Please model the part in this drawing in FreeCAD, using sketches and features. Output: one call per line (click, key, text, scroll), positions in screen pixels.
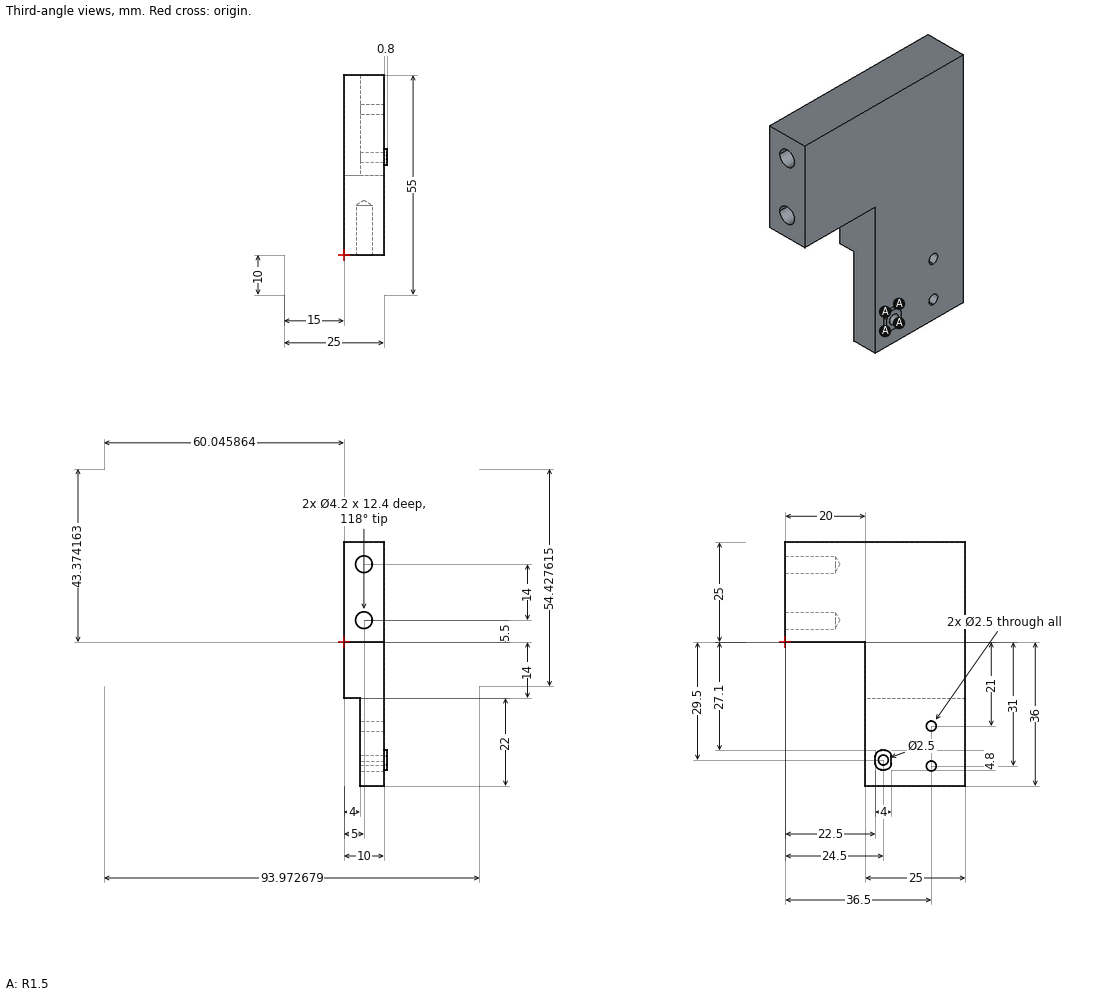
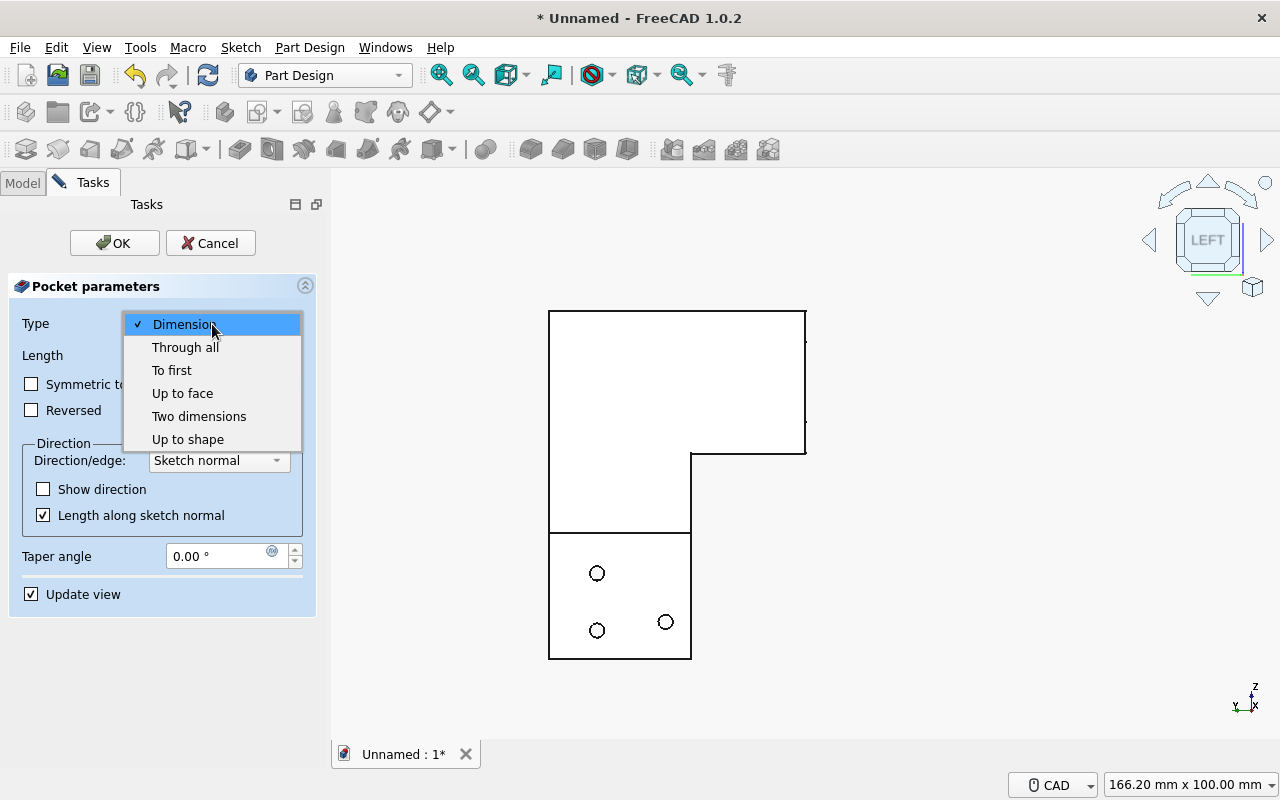
click(212, 348)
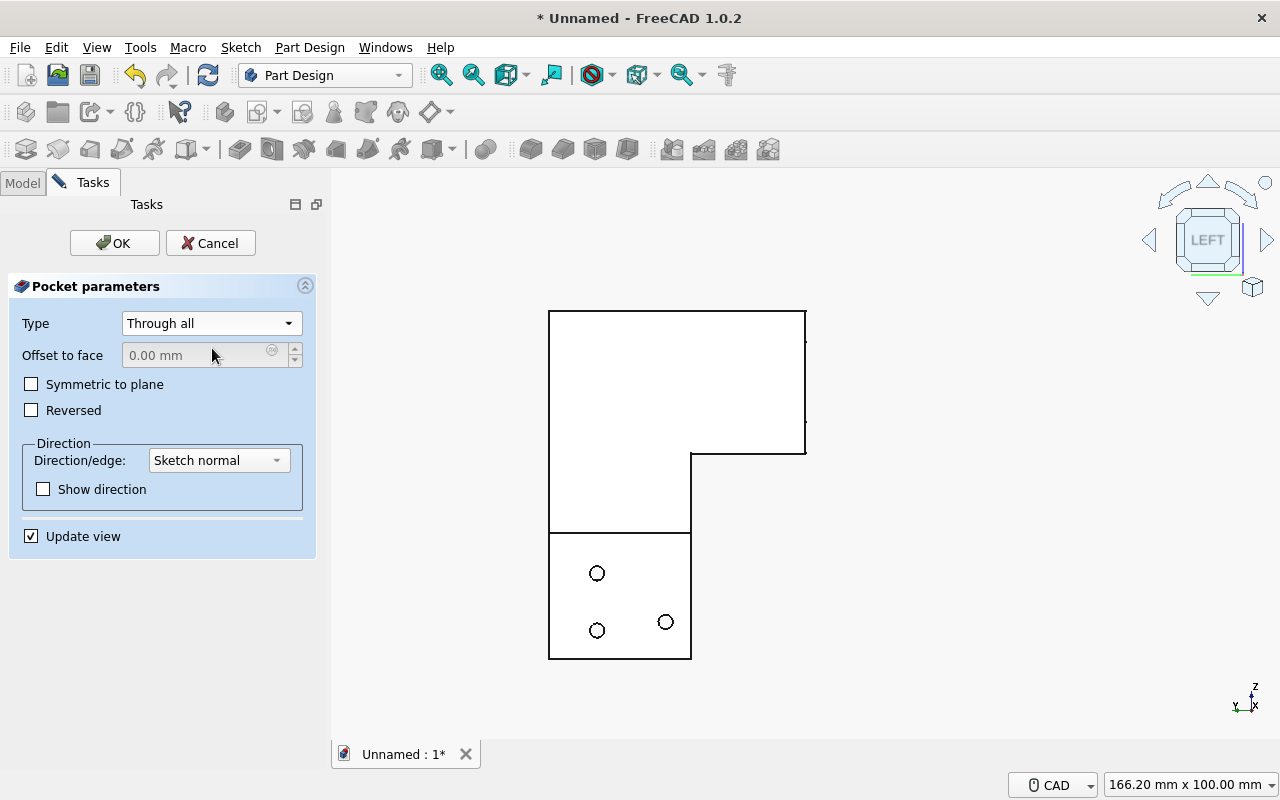
click(115, 243)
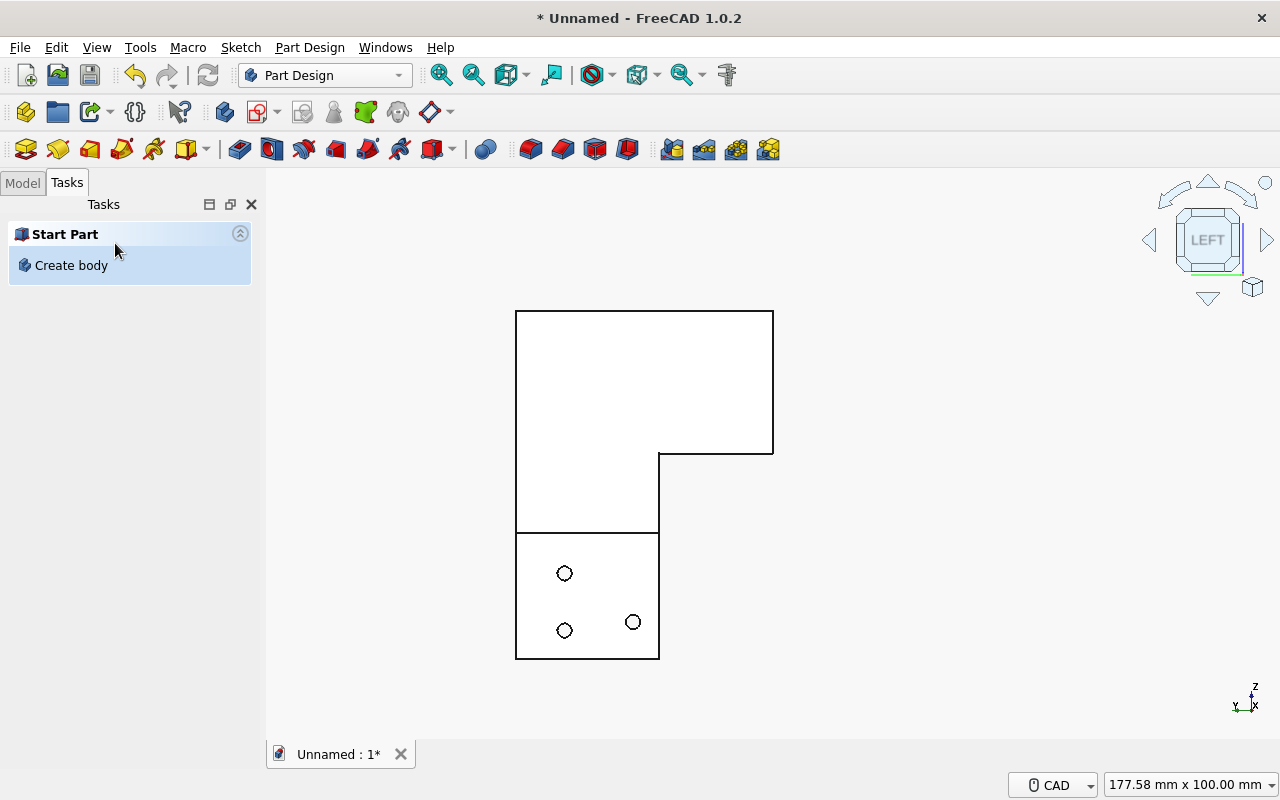
scroll(645, 635, up, 11)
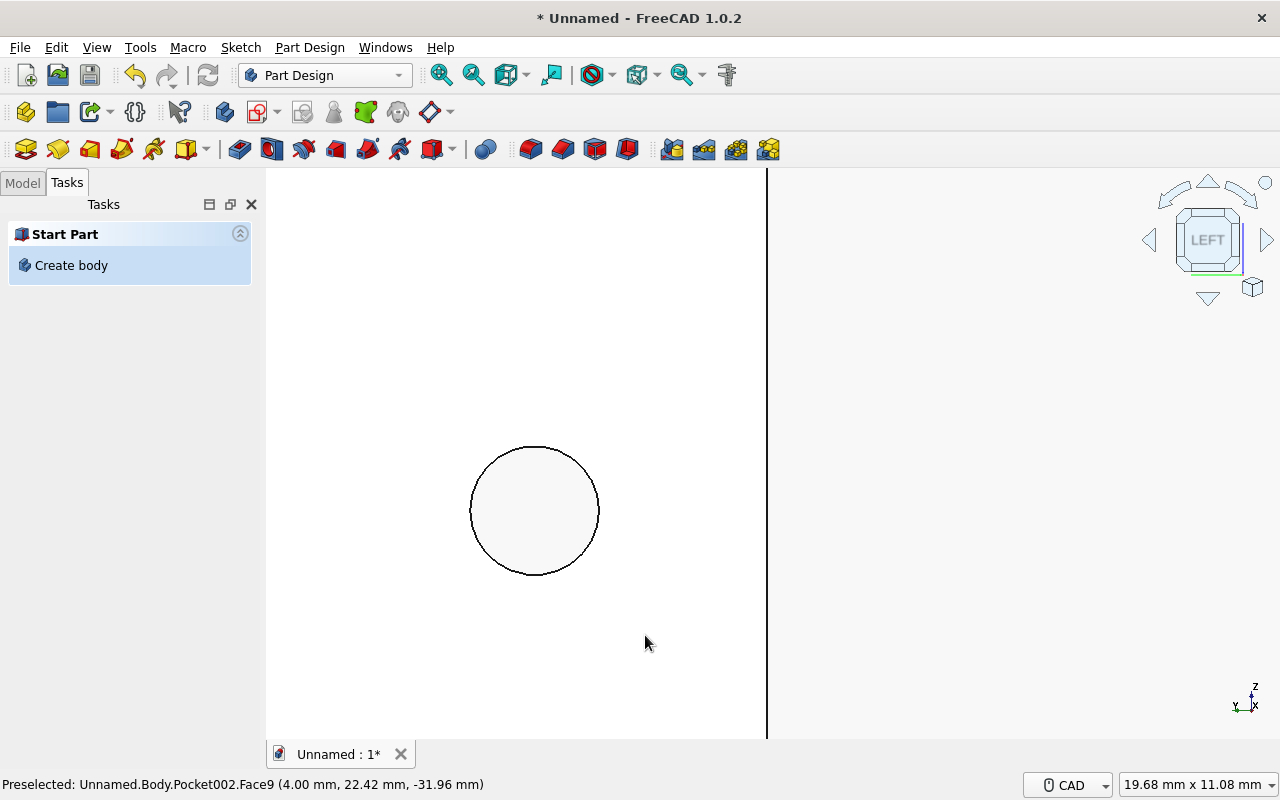
click(442, 76)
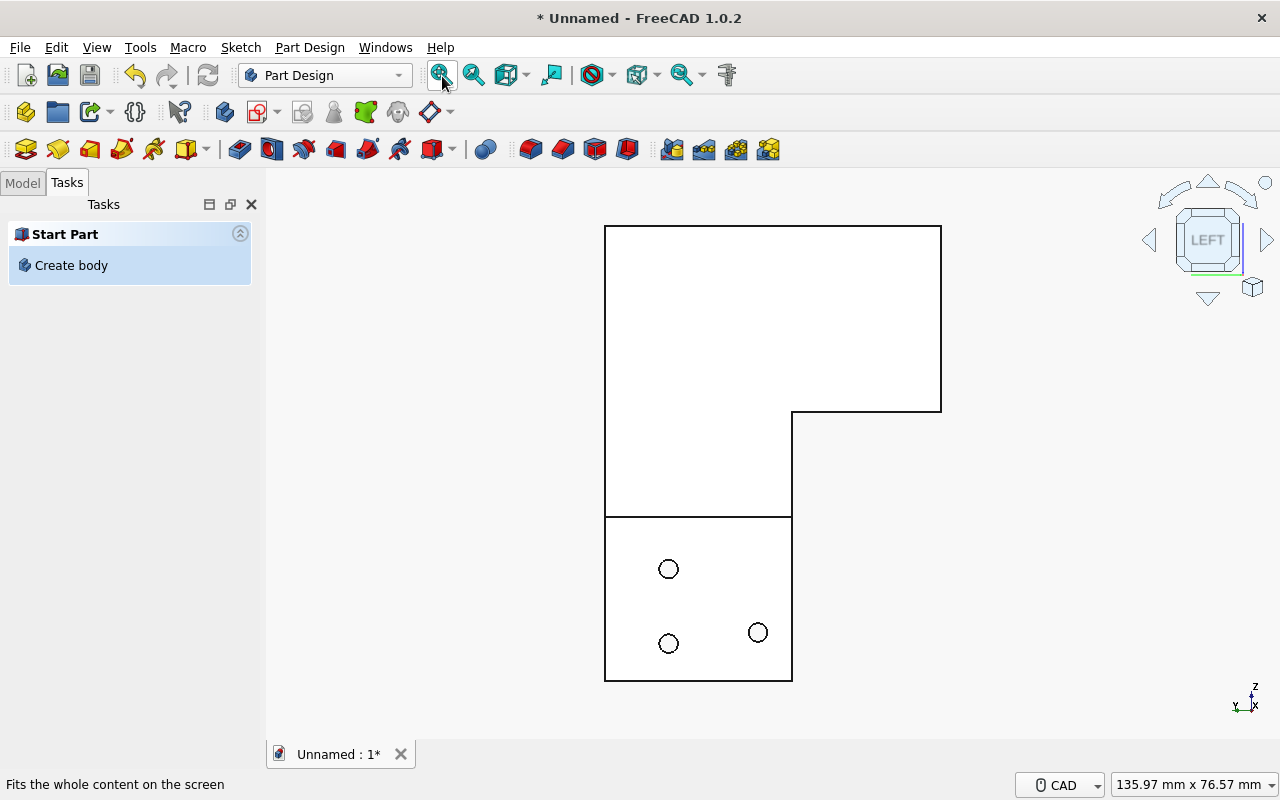
key(0)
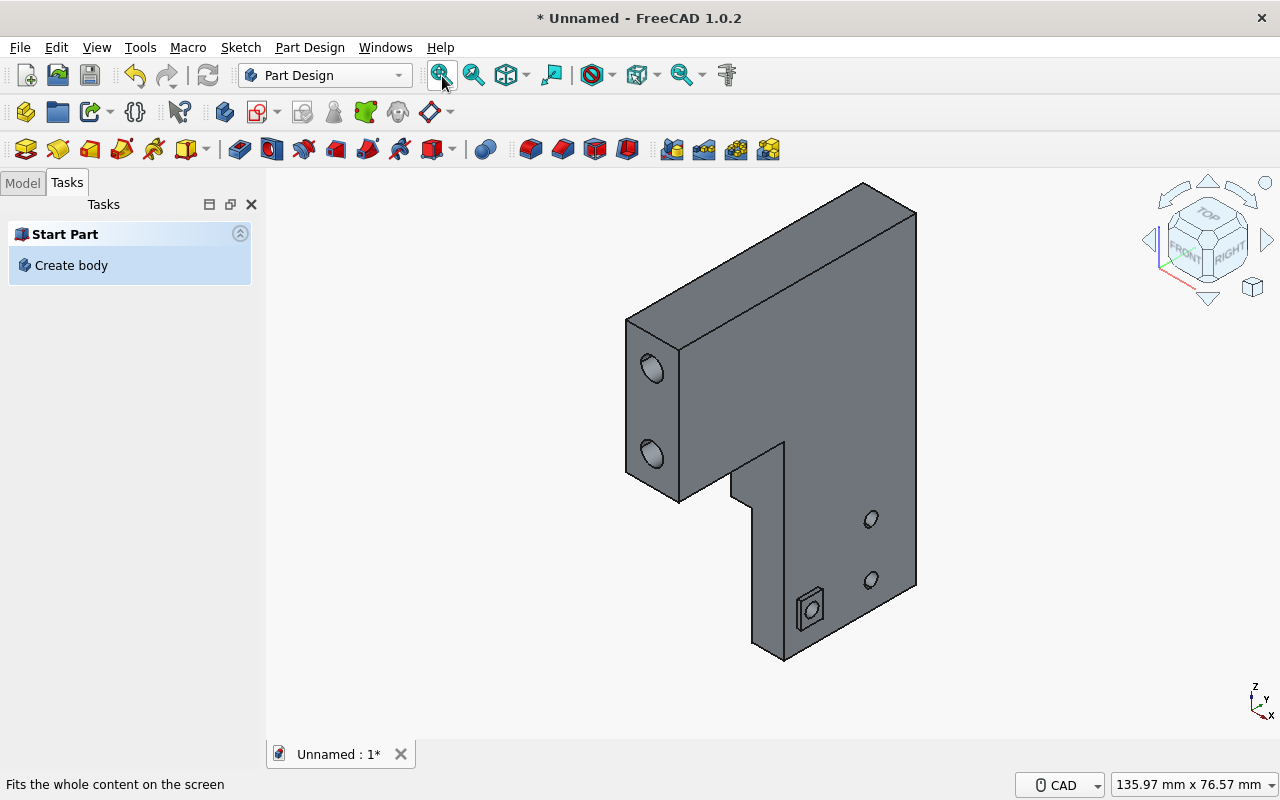
scroll(799, 628, up, 10)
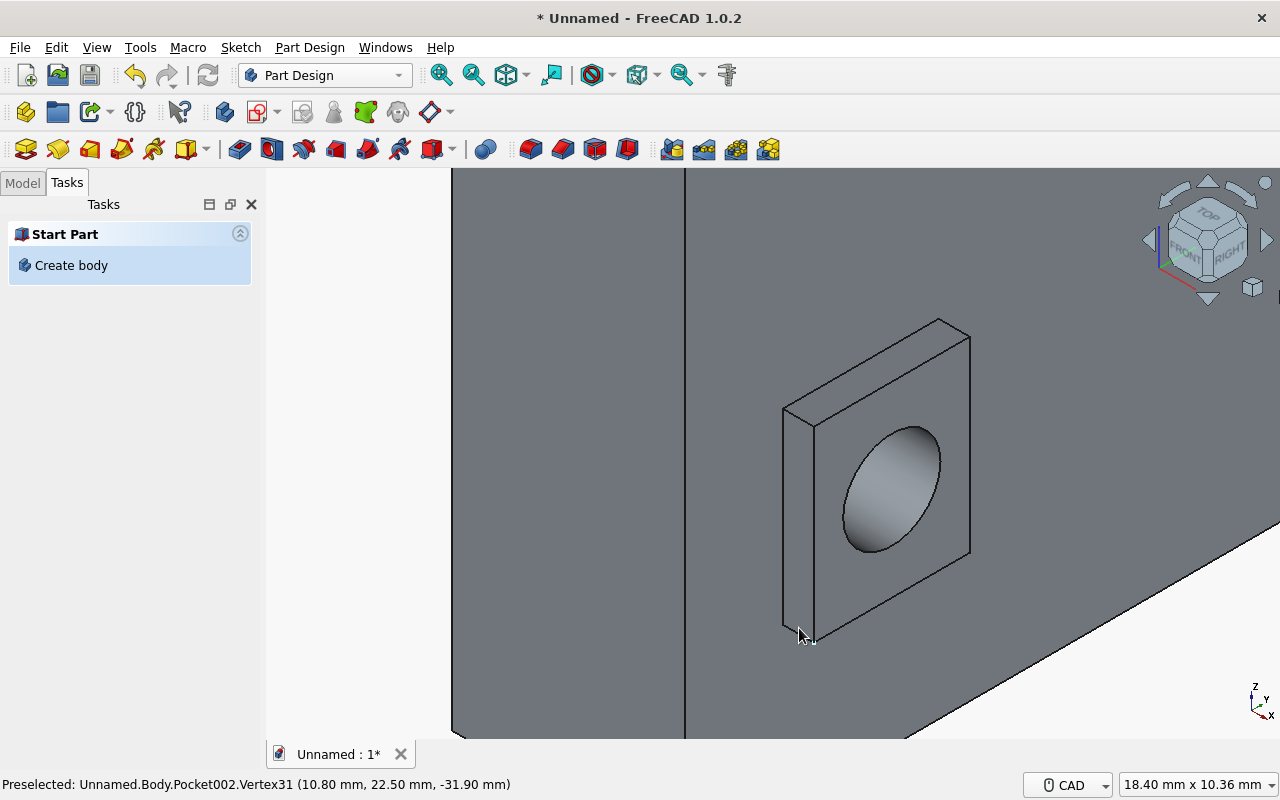
click(798, 417)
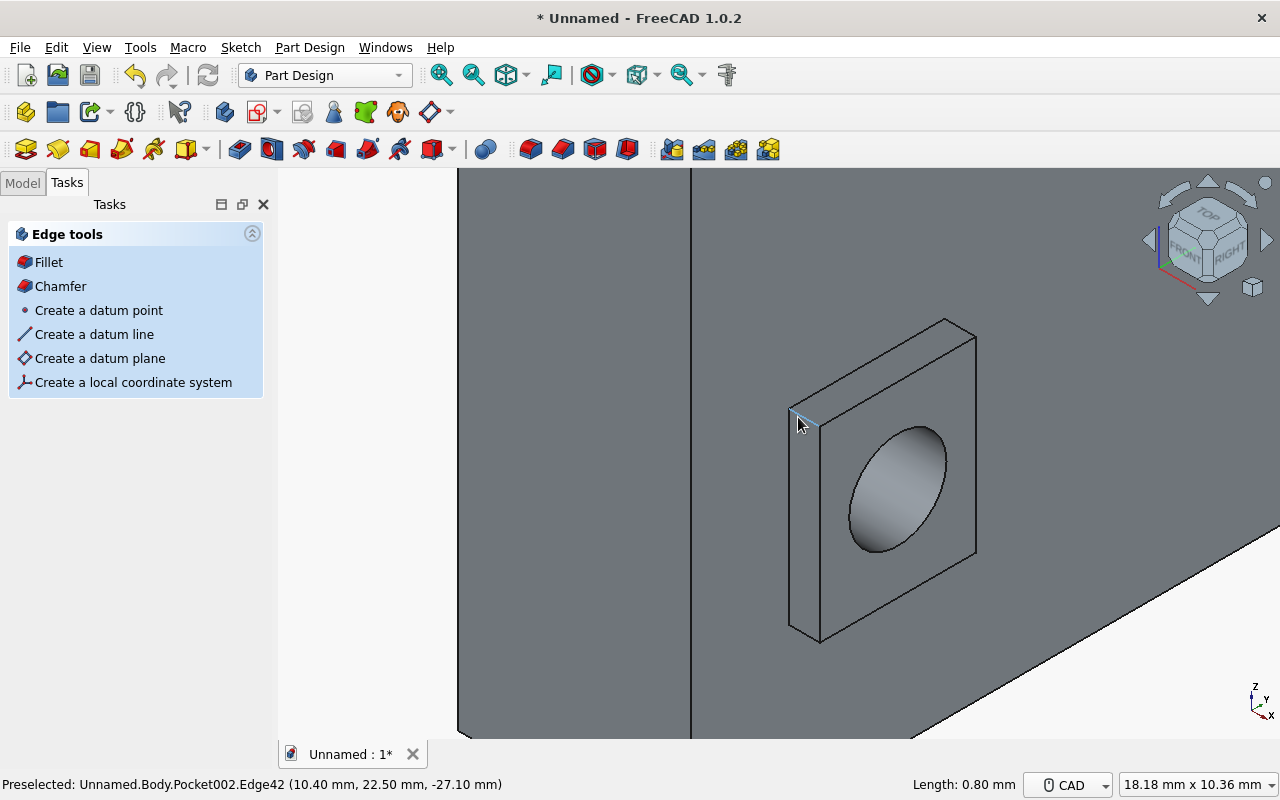
click(442, 76)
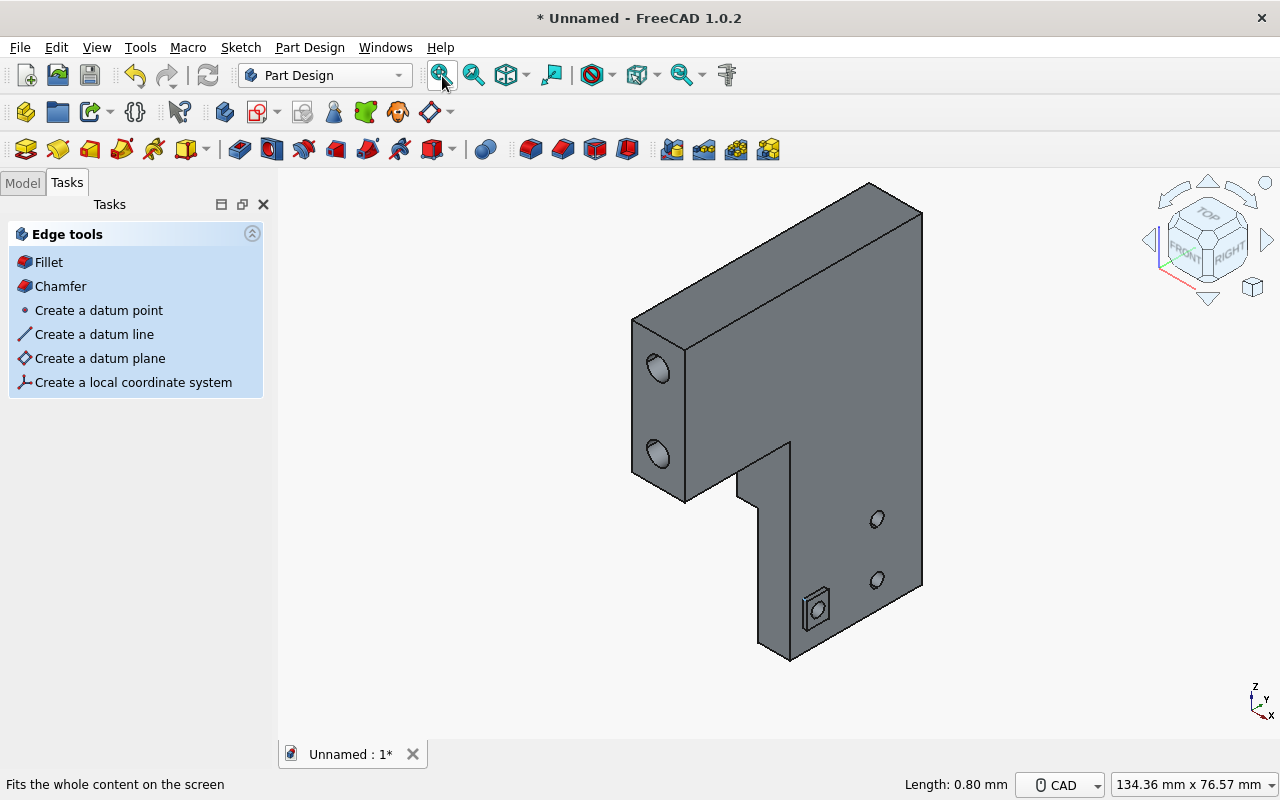
key(2)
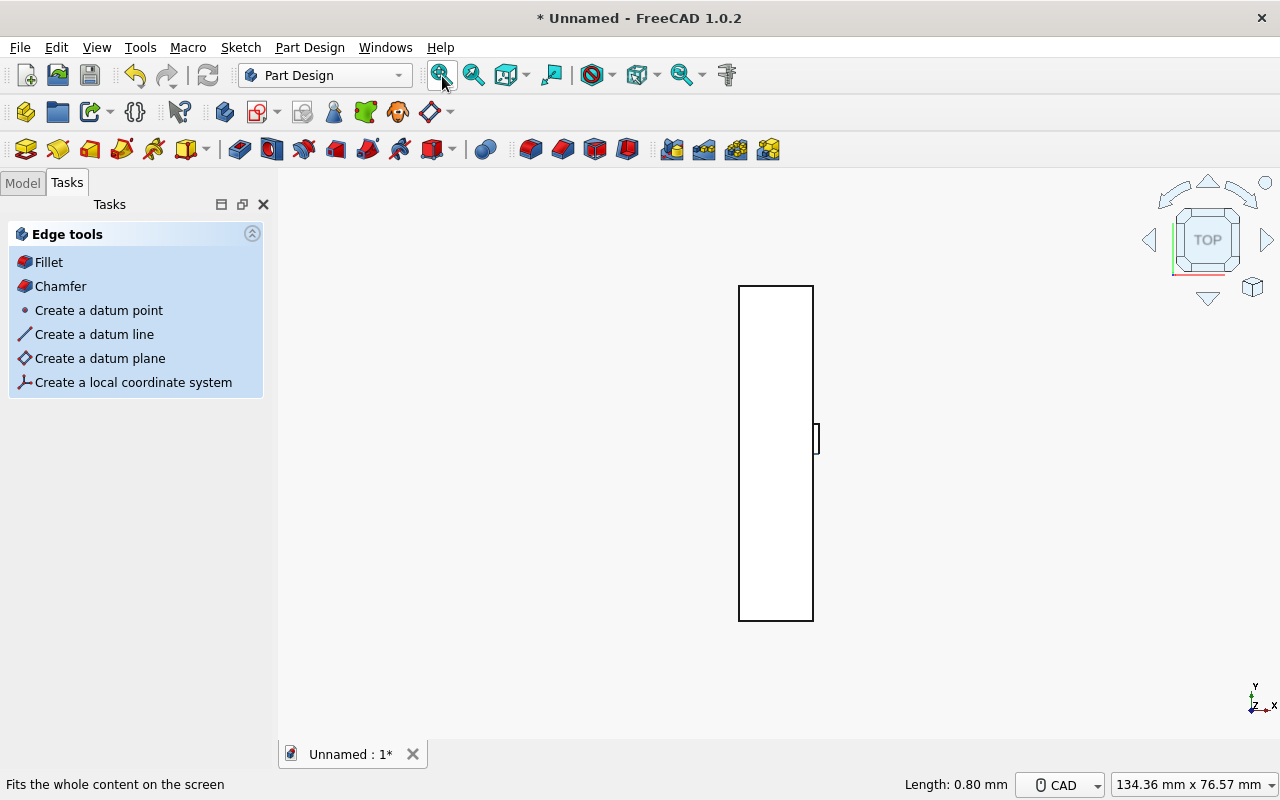
scroll(816, 452, up, 10)